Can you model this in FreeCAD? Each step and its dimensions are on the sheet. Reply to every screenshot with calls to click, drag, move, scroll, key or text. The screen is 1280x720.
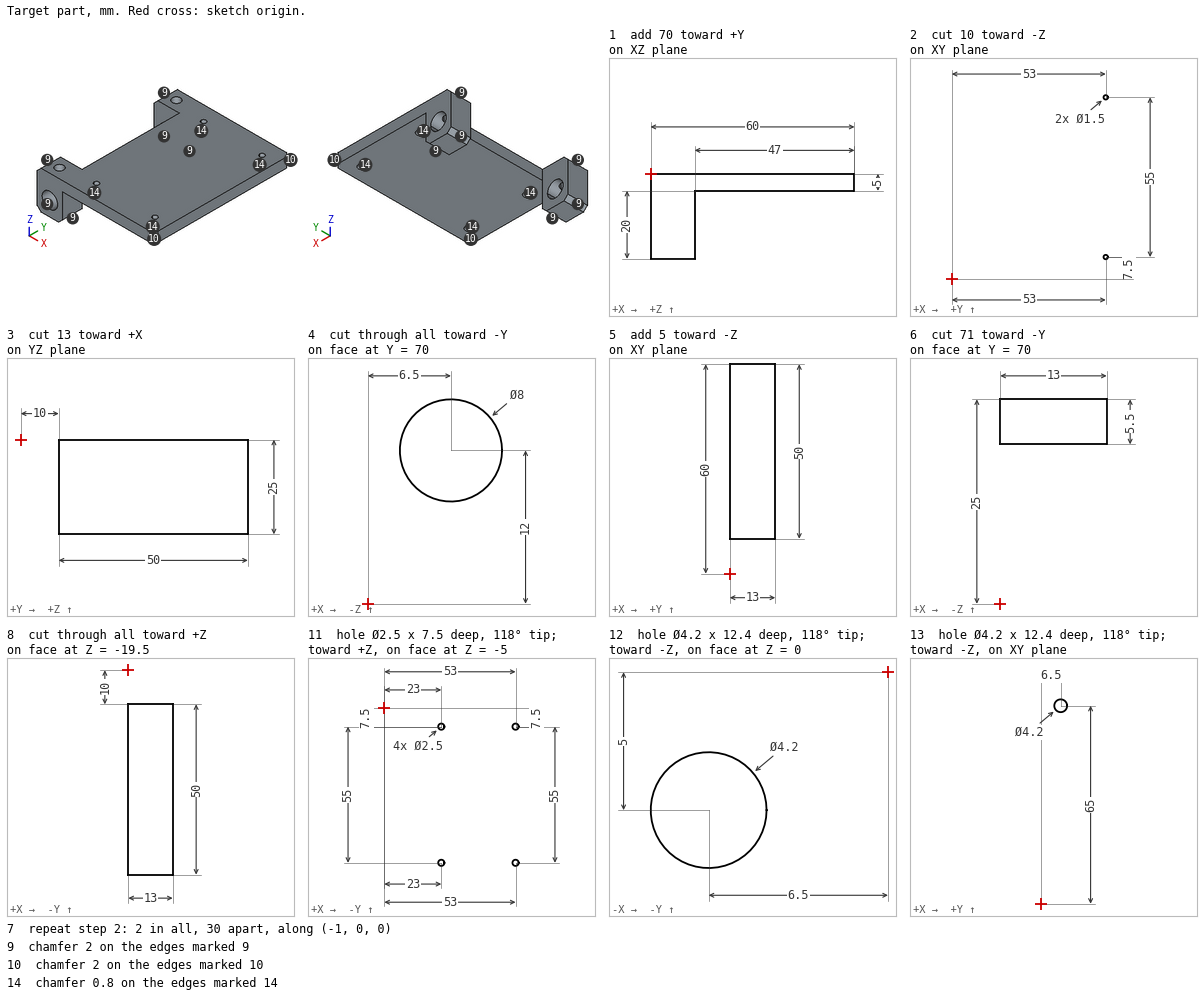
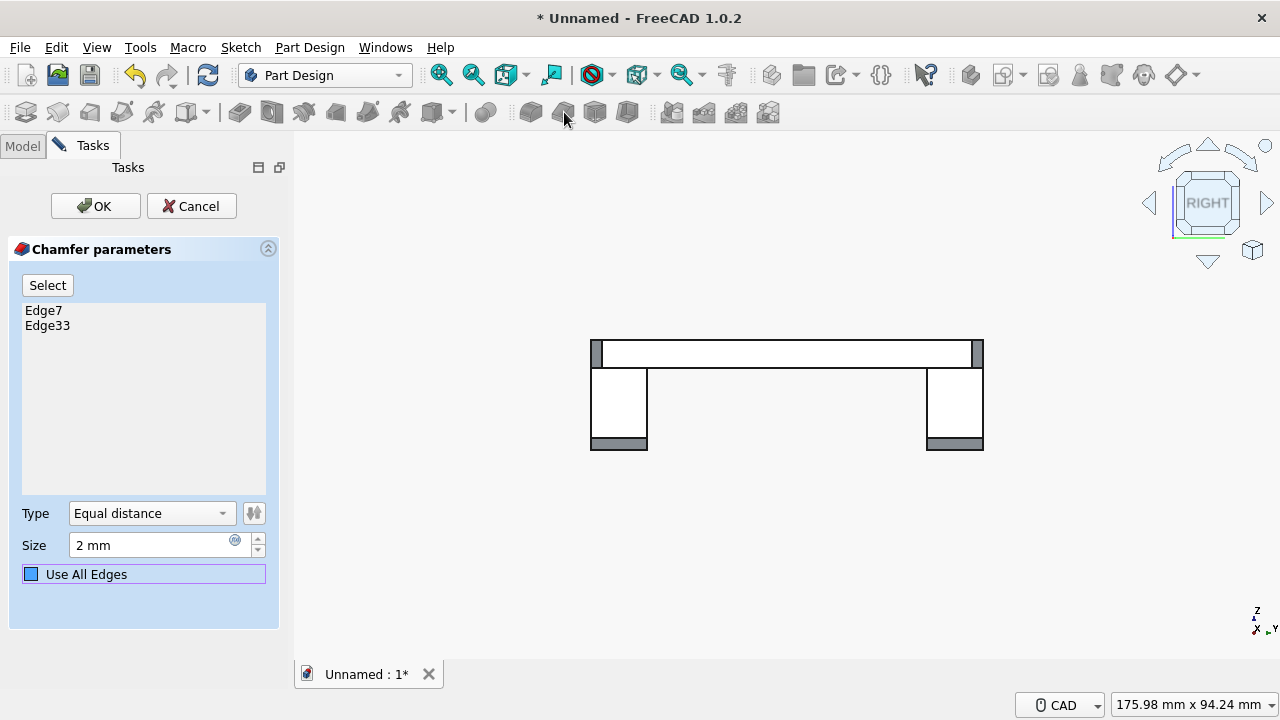
click(96, 206)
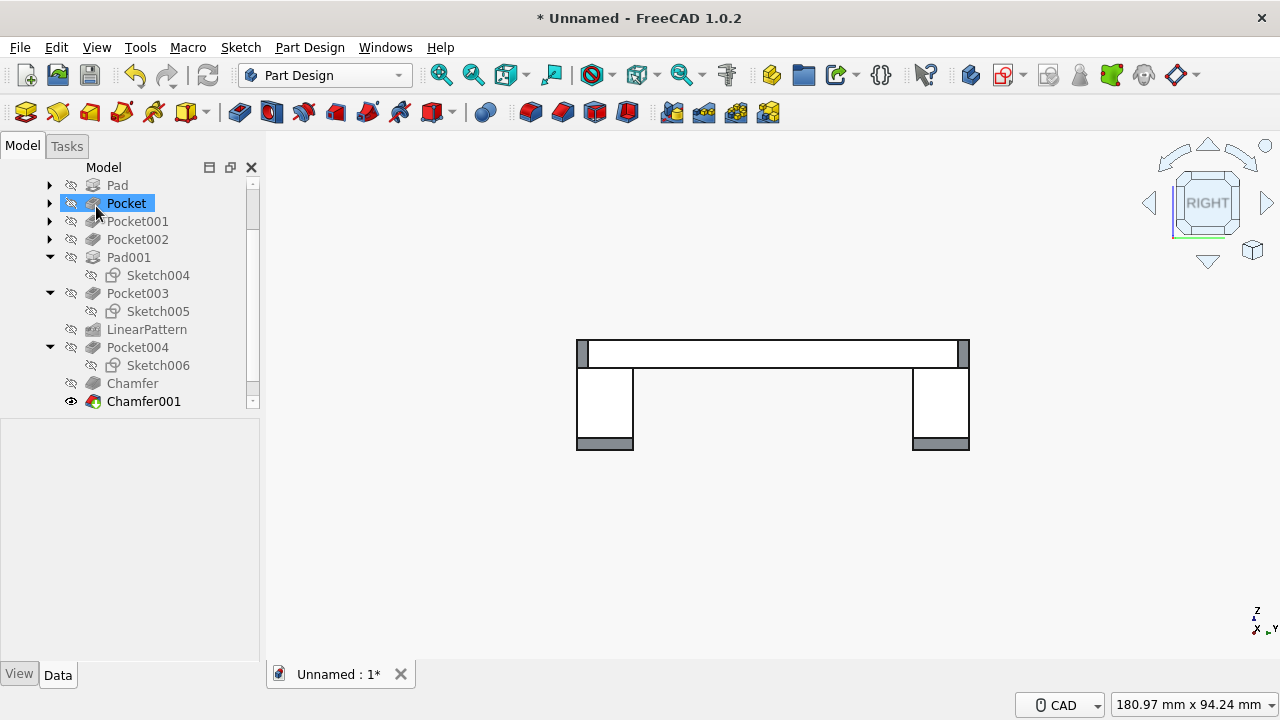
key(v)
key(f)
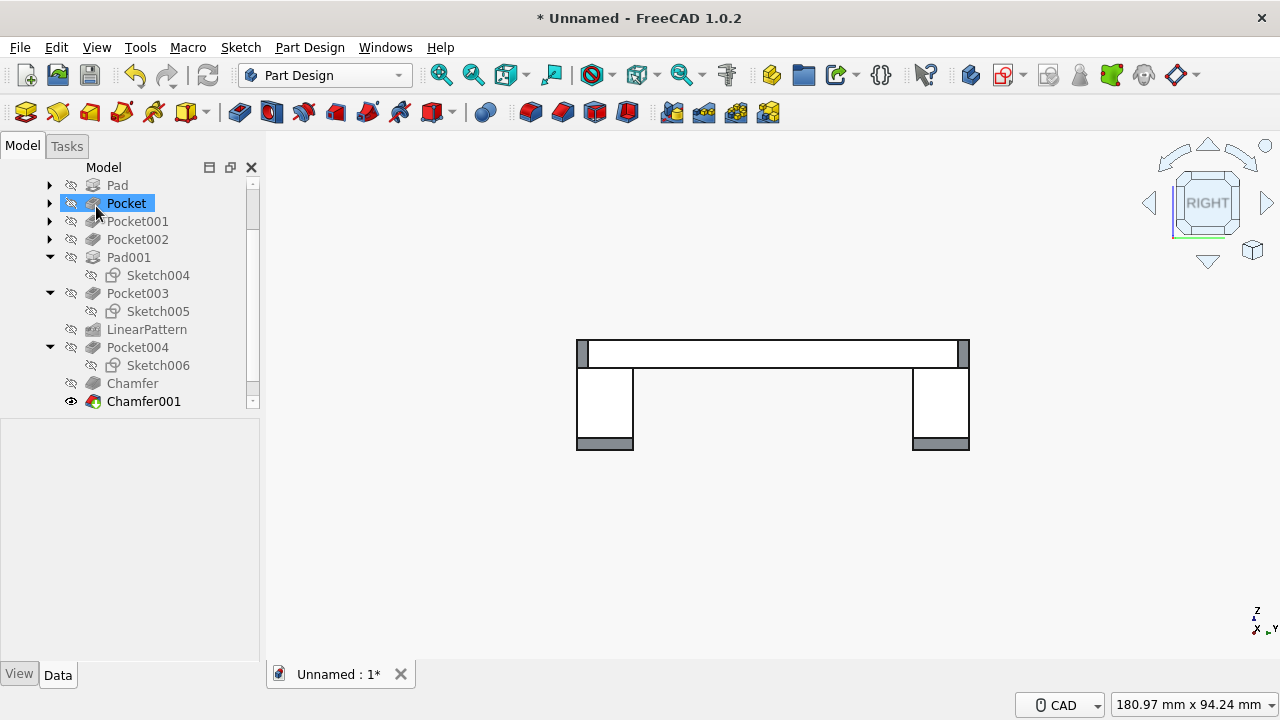
key(5)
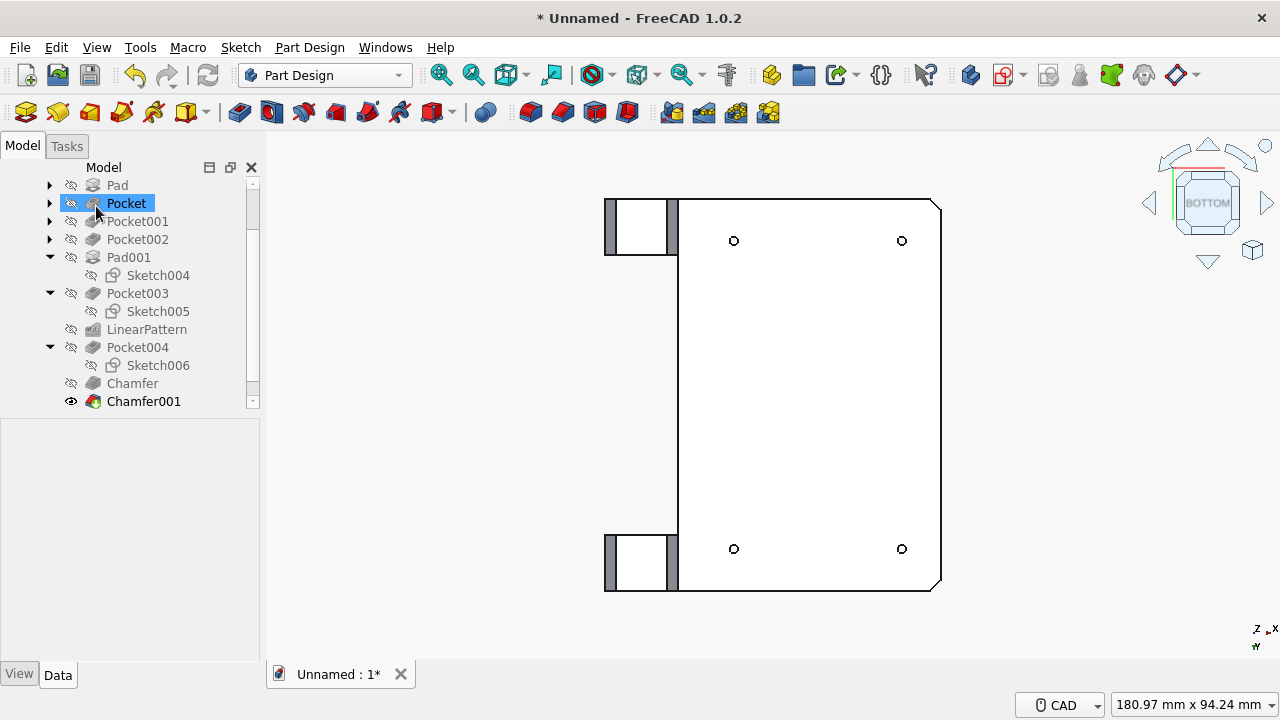
click(809, 394)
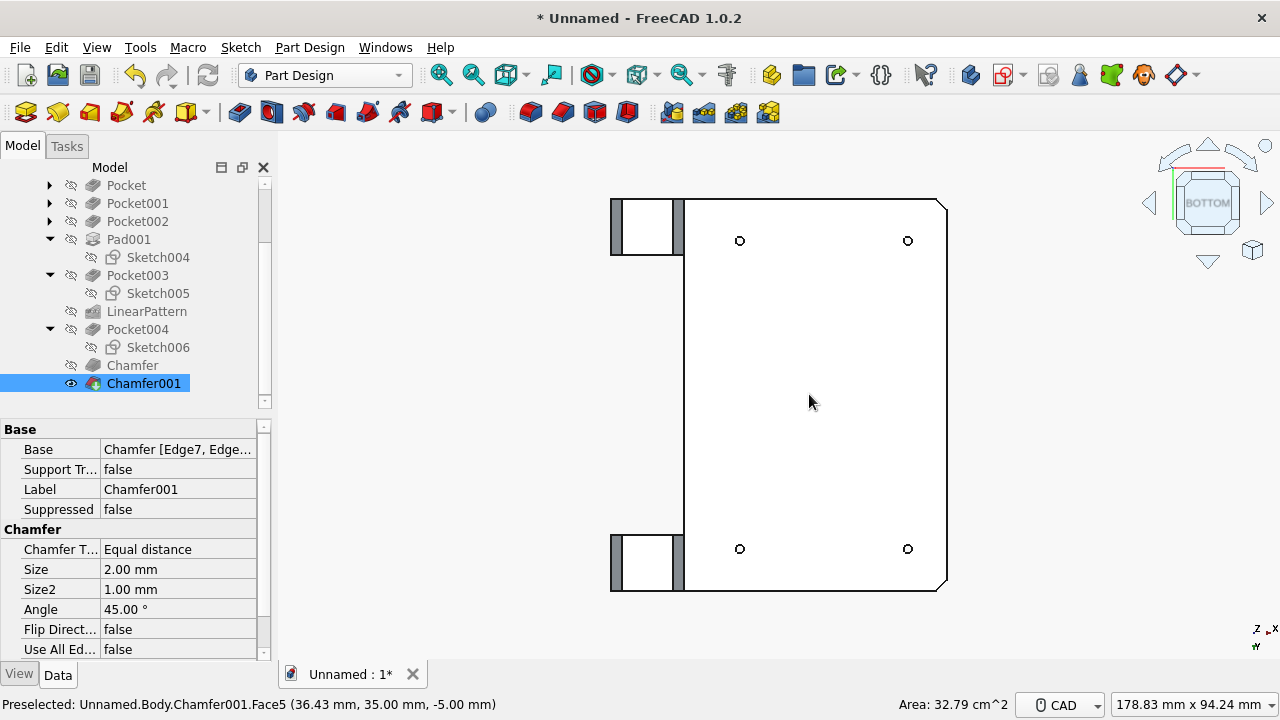
click(1004, 76)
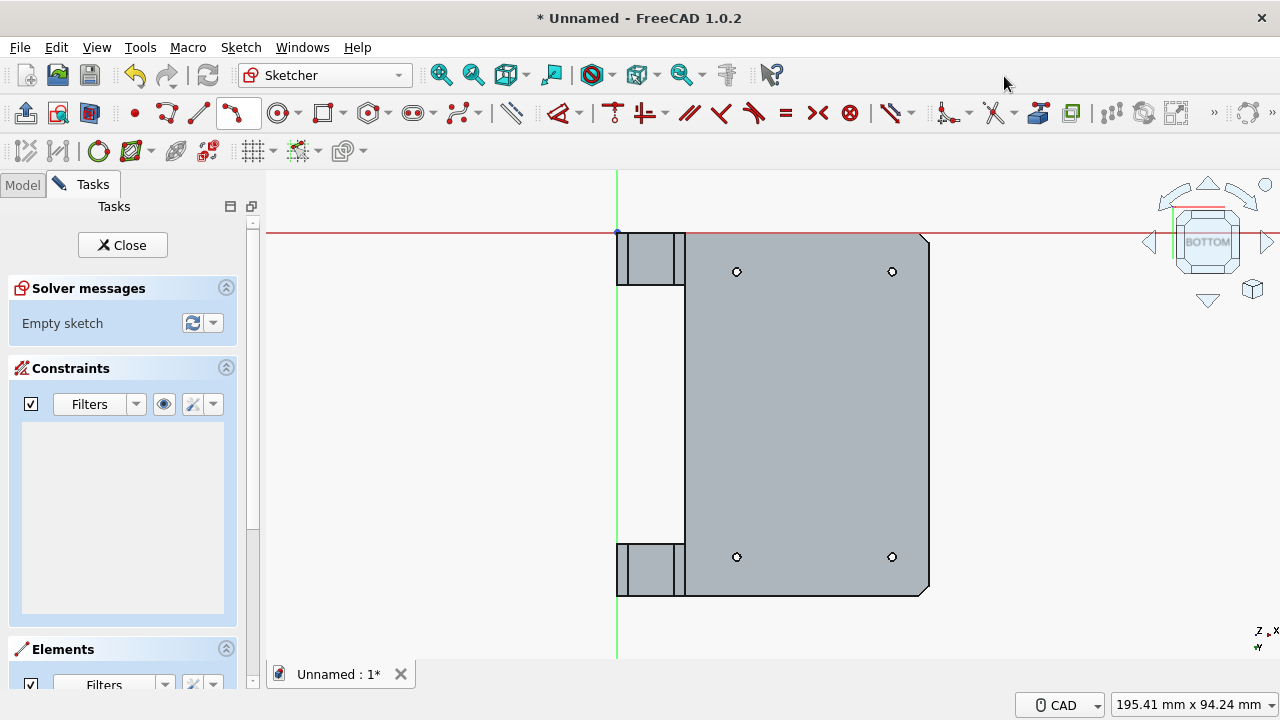
click(278, 114)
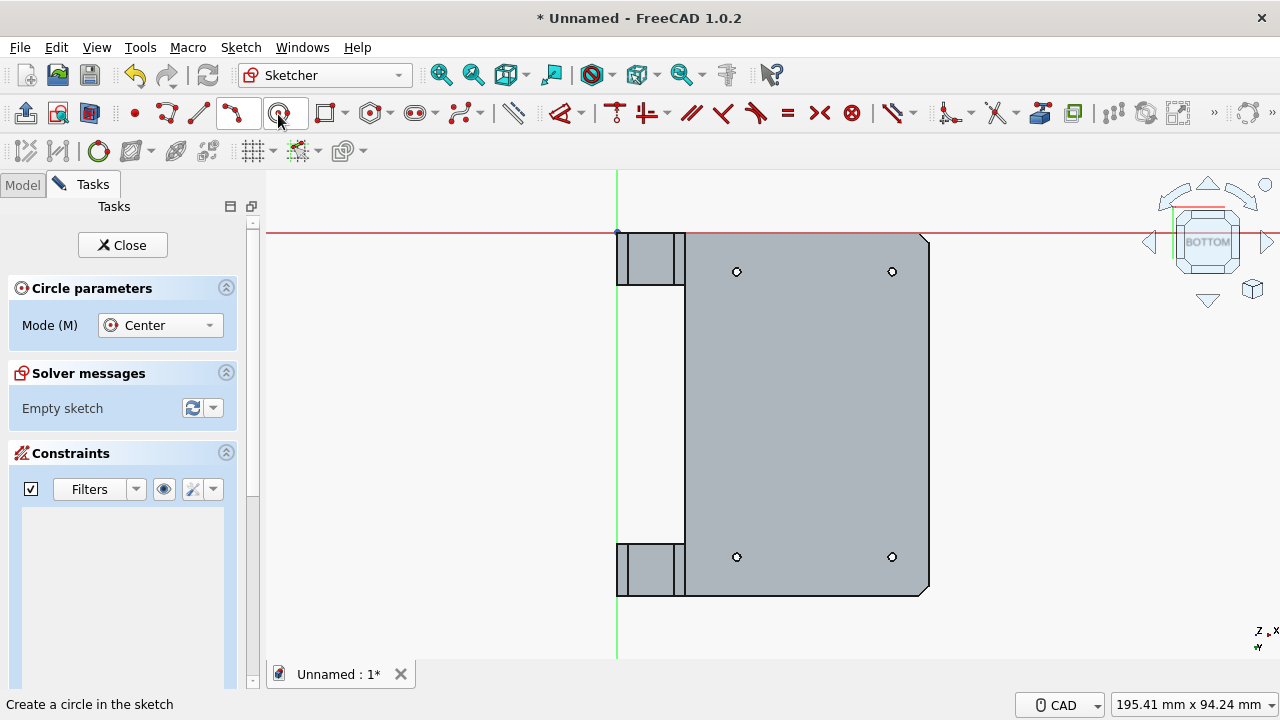
scroll(737, 272, up, 7)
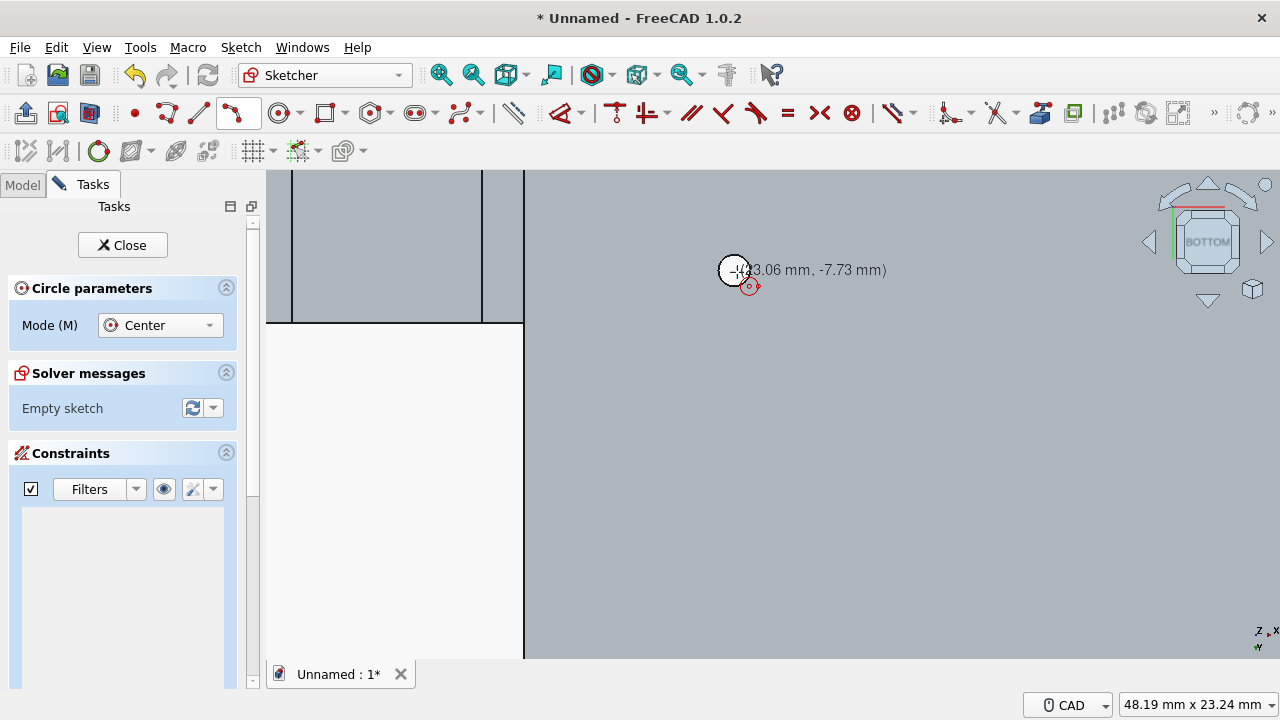
scroll(666, 294, down, 7)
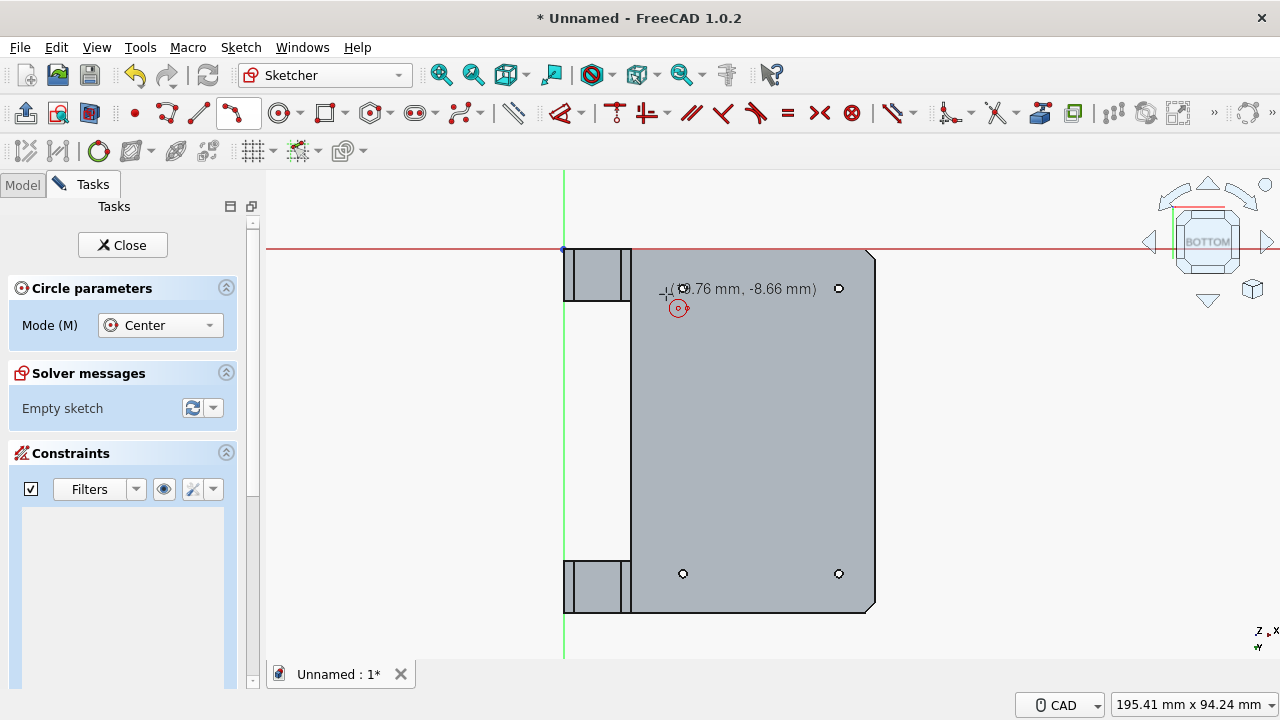
click(683, 288)
move(688, 284)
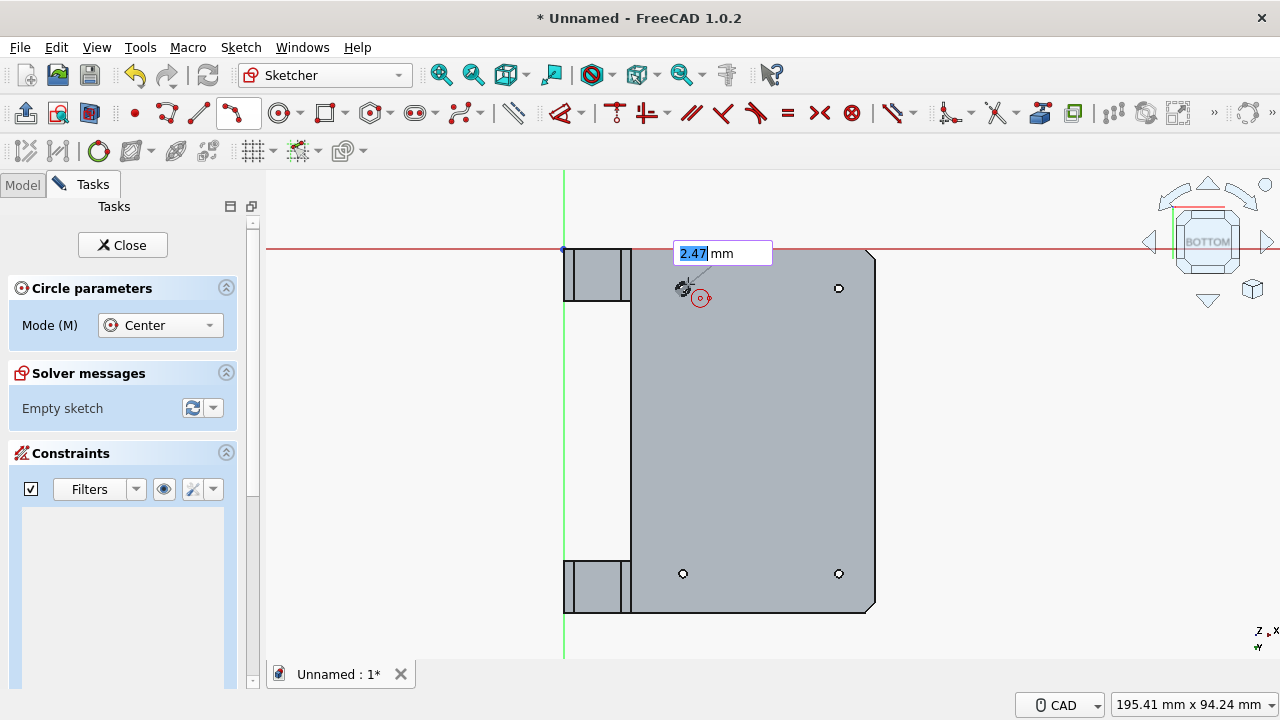
text(2.5)
key(Return)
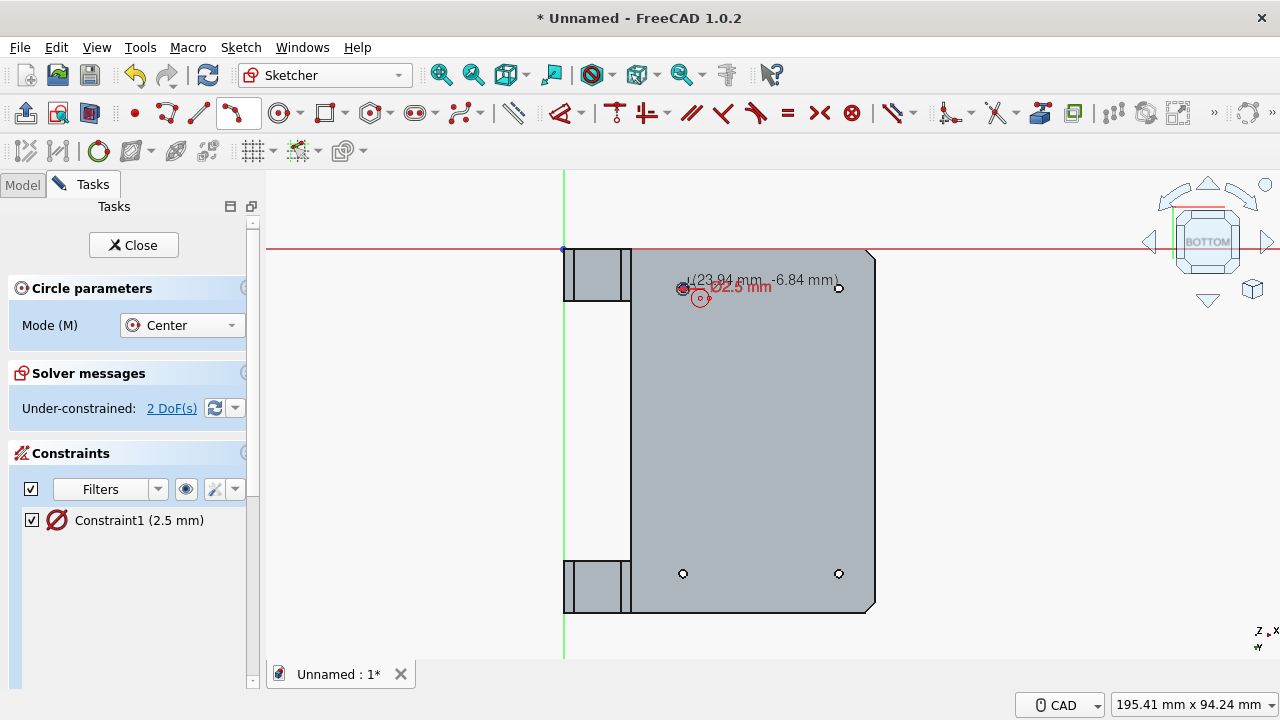
scroll(839, 288, up, 7)